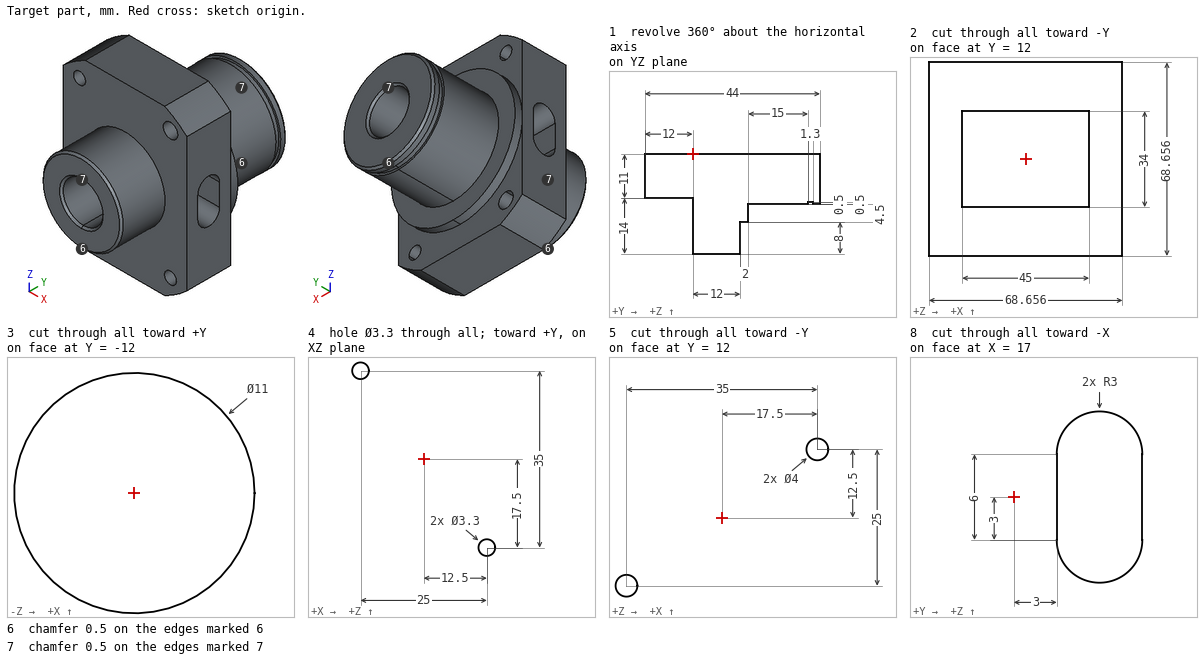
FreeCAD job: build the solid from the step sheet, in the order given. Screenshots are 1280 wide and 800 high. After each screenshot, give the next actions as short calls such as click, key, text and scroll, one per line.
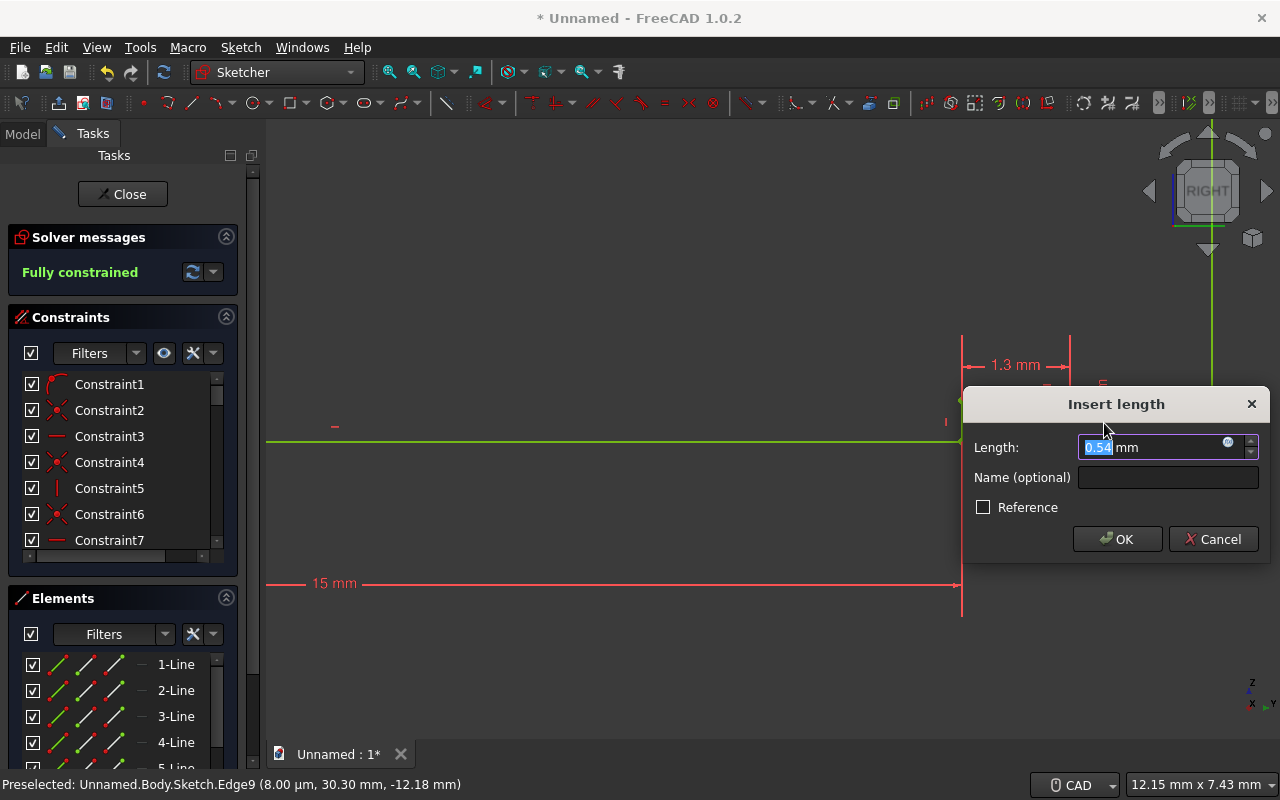
text(0.5)
key(Return)
key(Escape)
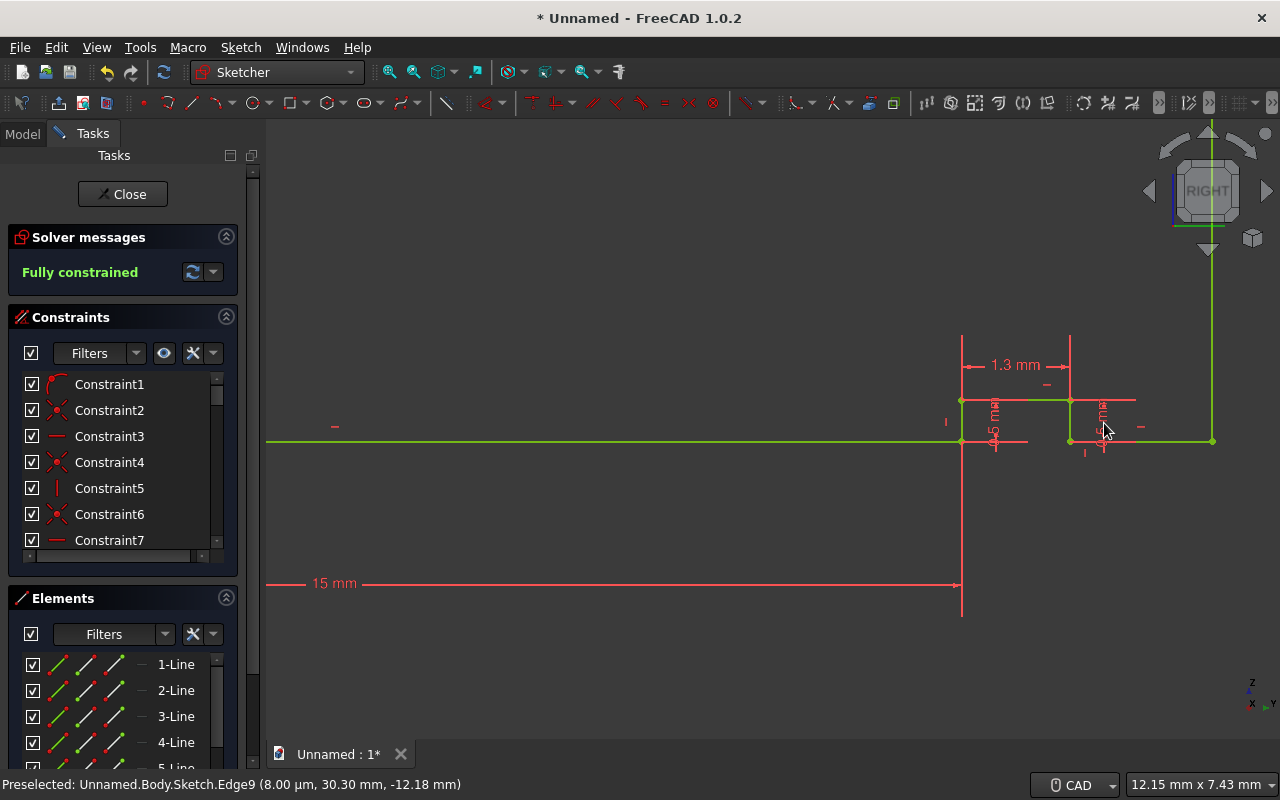
click(123, 194)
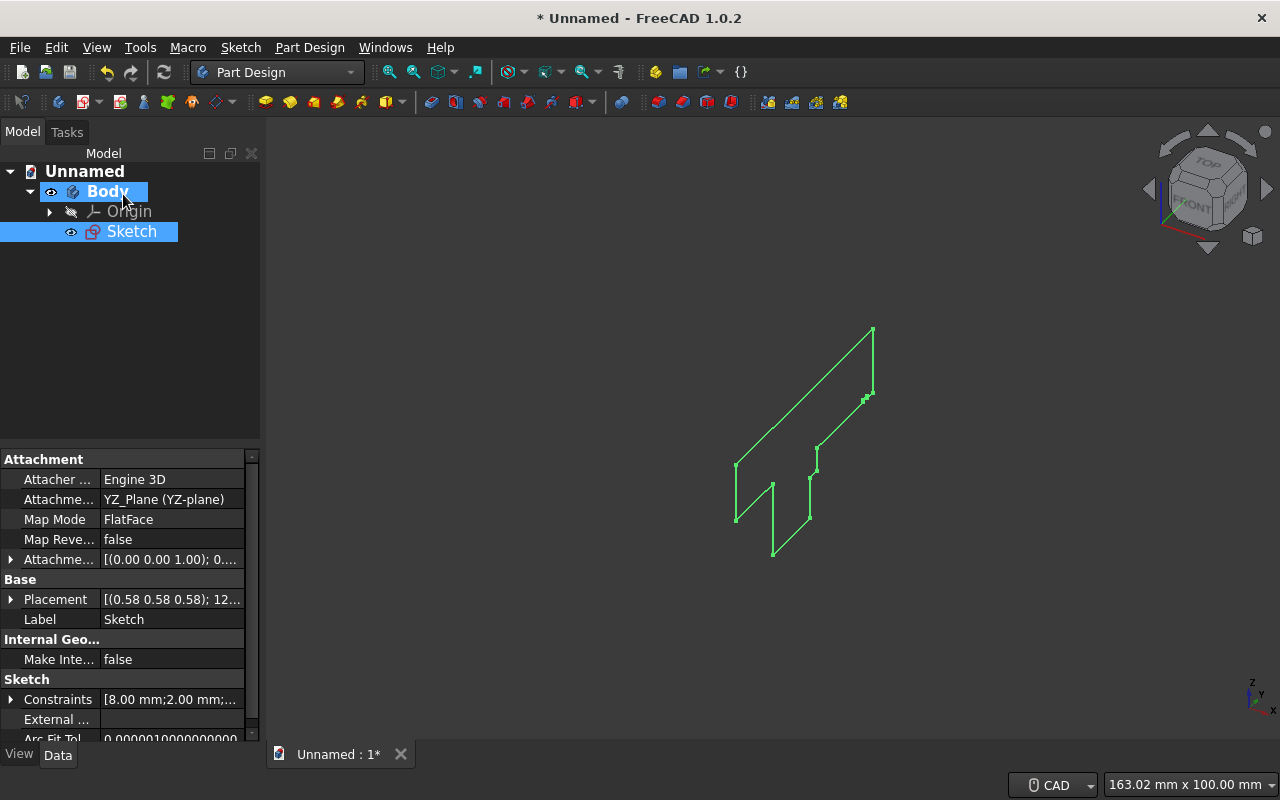
click(290, 102)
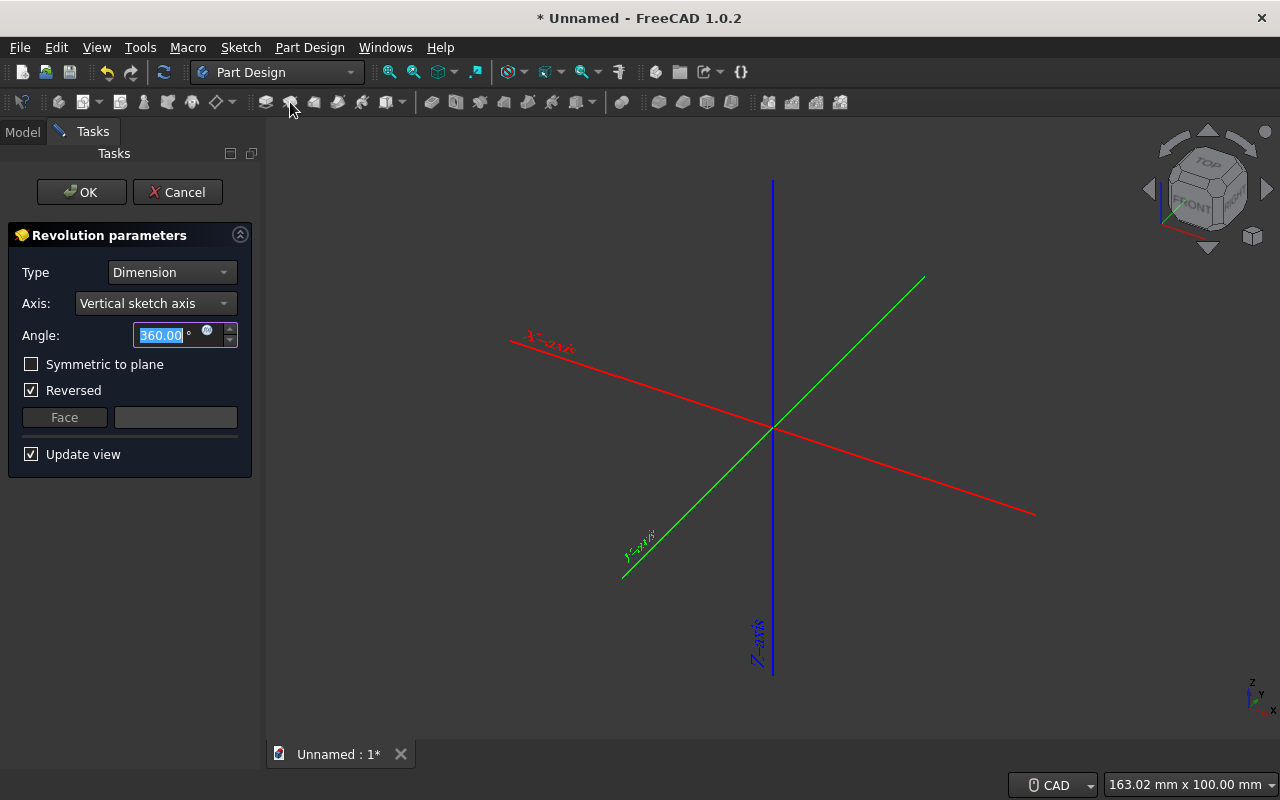
click(156, 304)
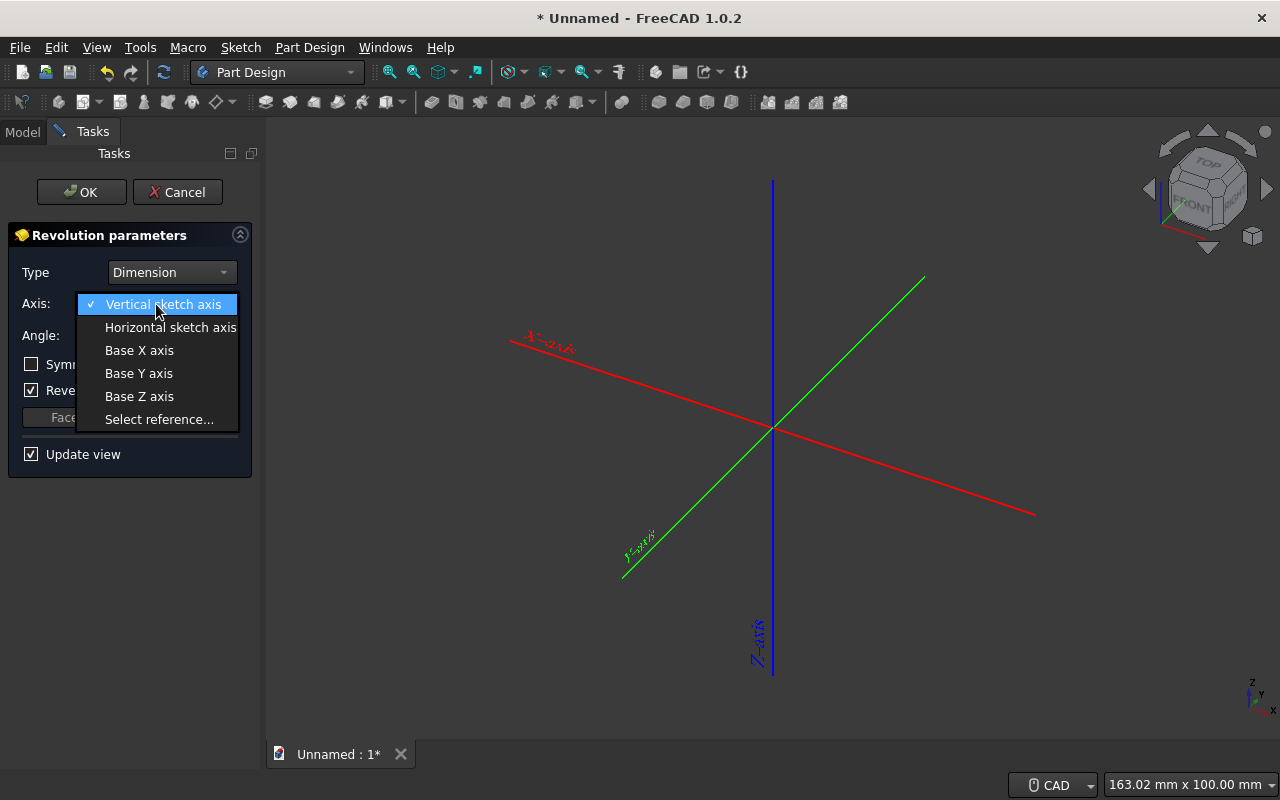
click(156, 328)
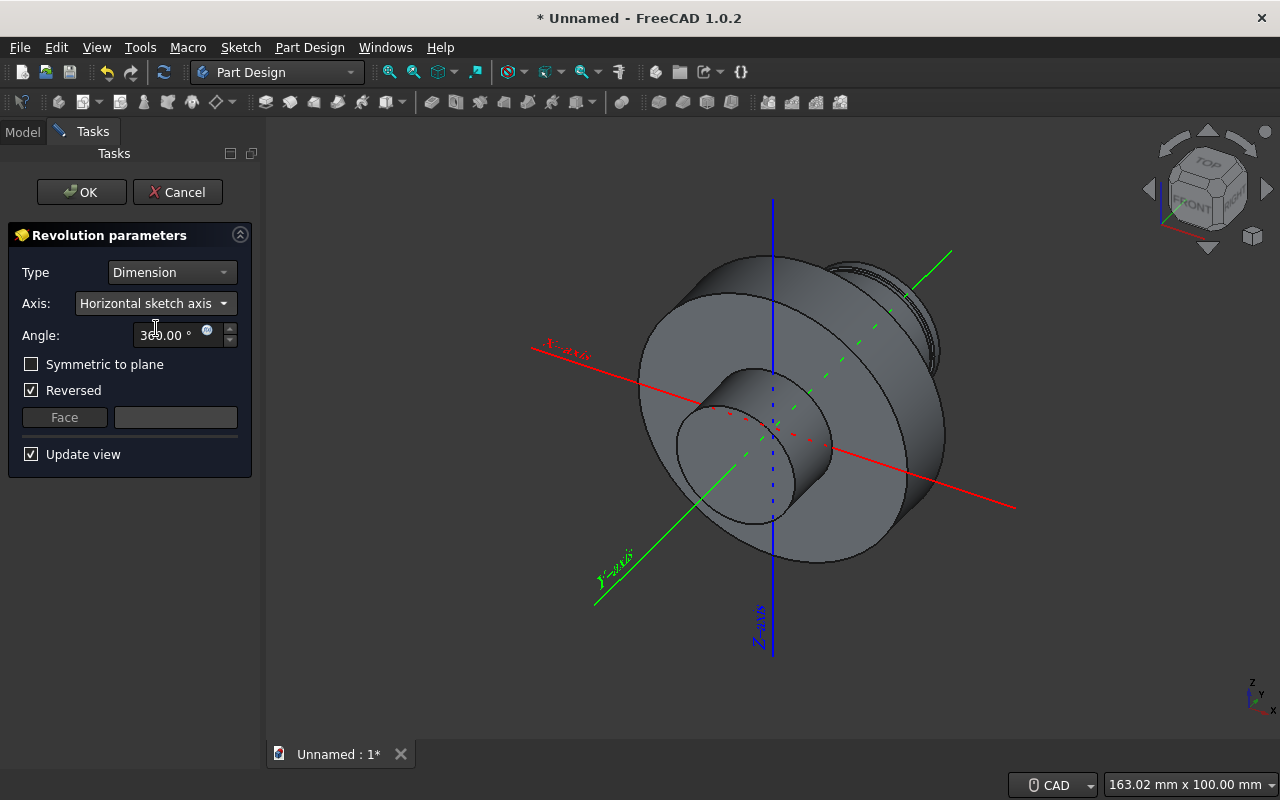
click(82, 192)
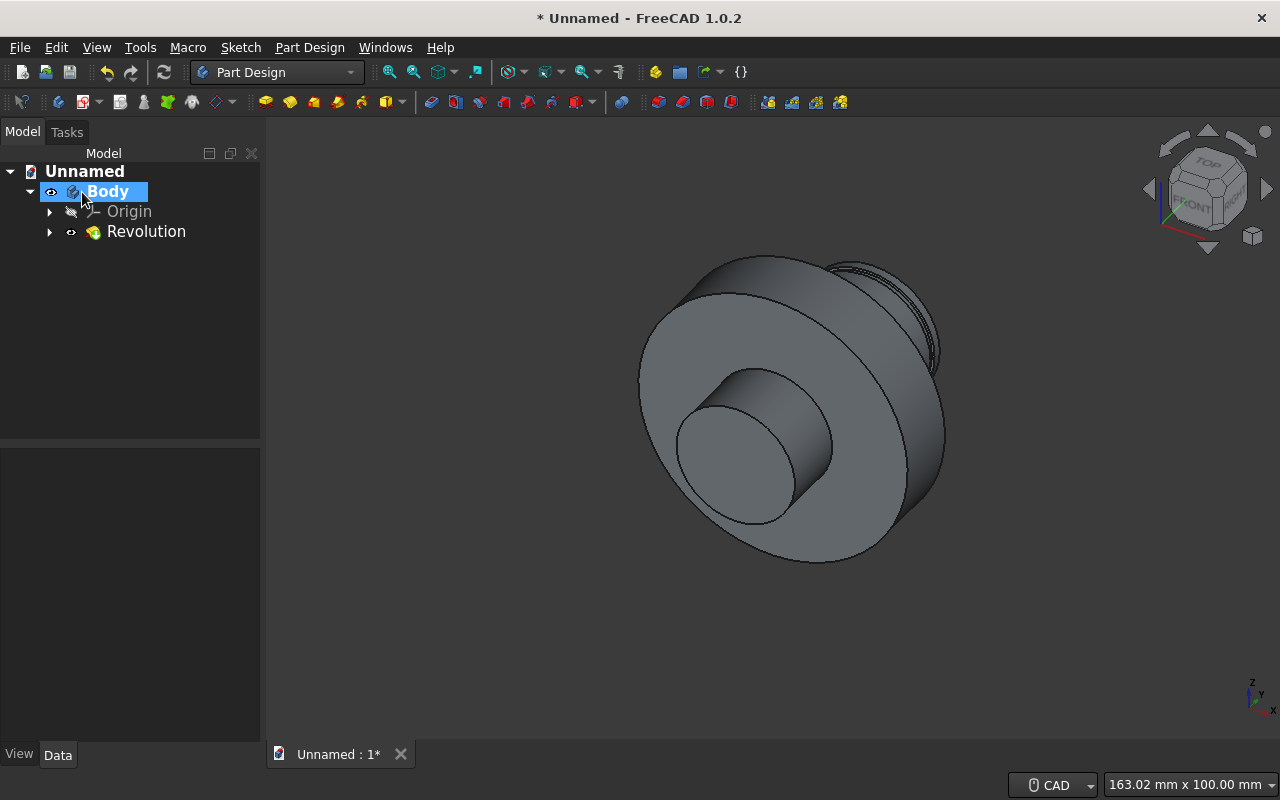
key(4)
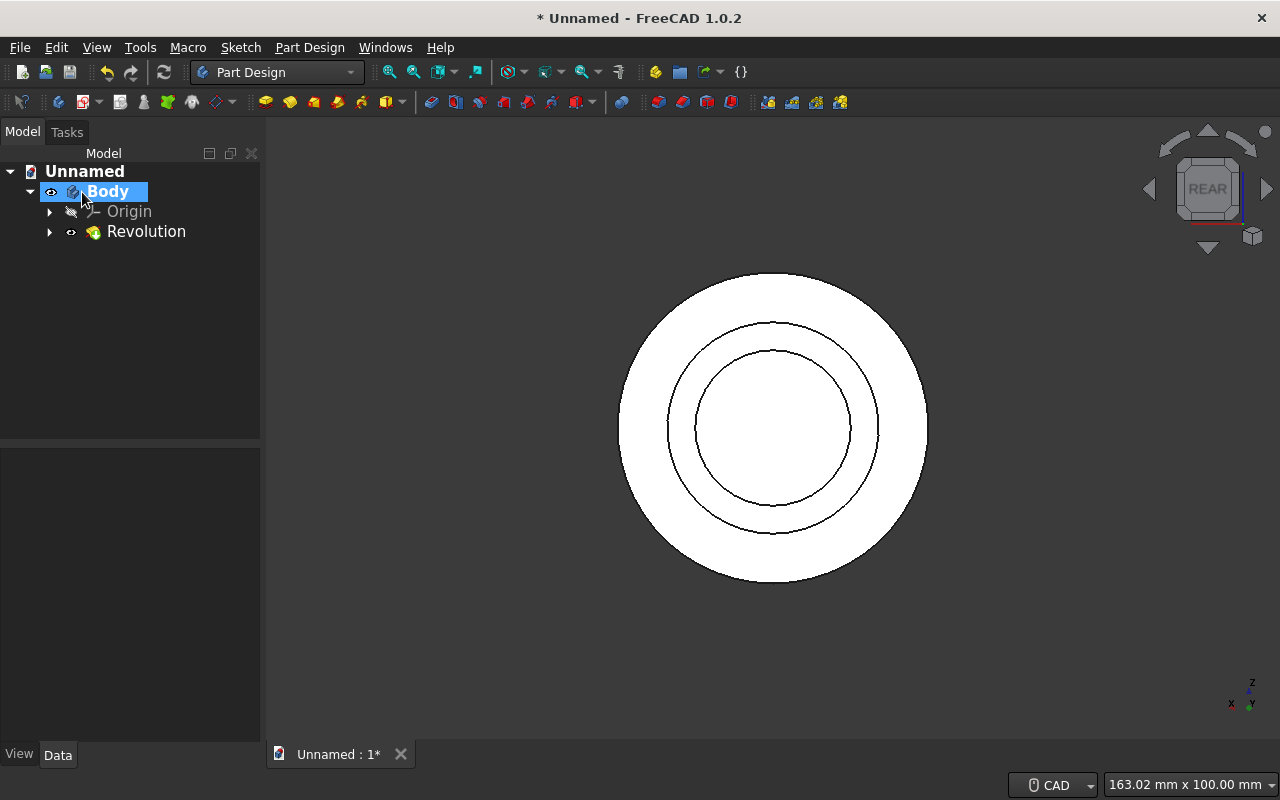
click(773, 294)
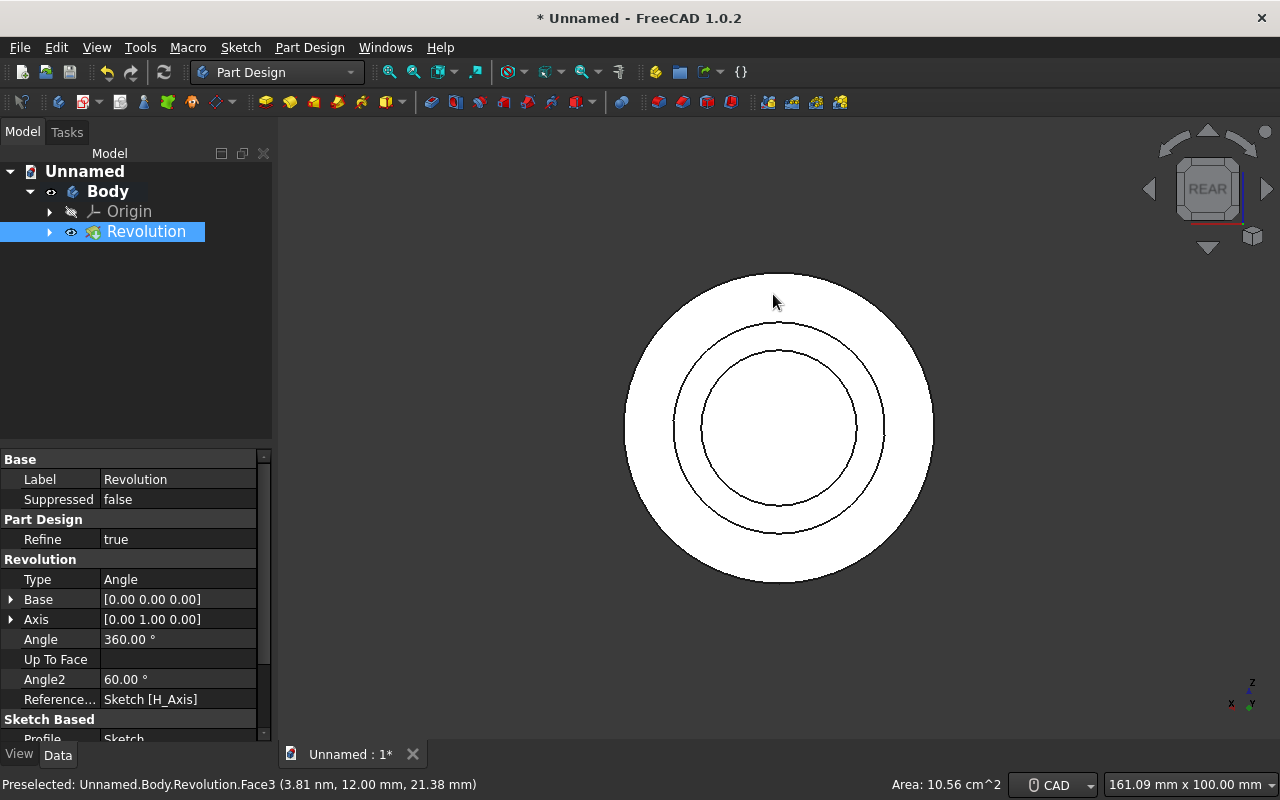
click(84, 102)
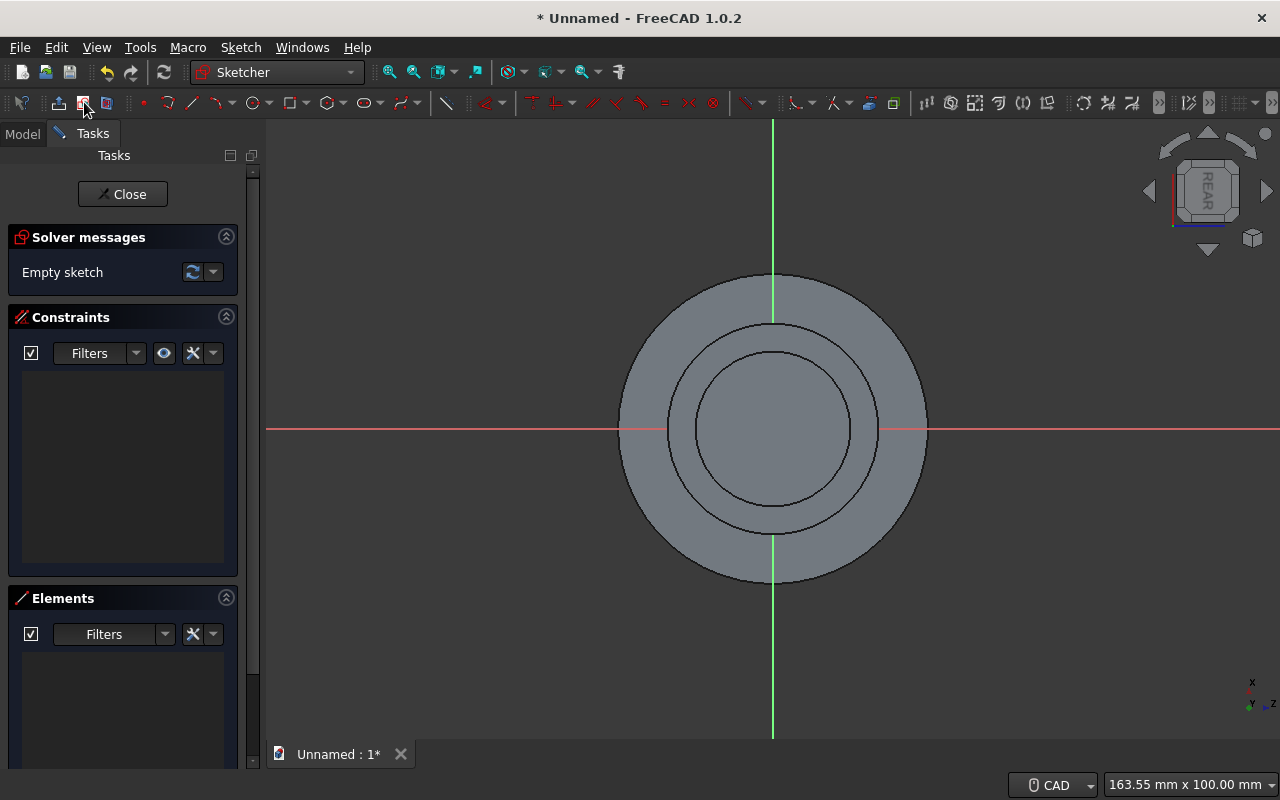
click(108, 104)